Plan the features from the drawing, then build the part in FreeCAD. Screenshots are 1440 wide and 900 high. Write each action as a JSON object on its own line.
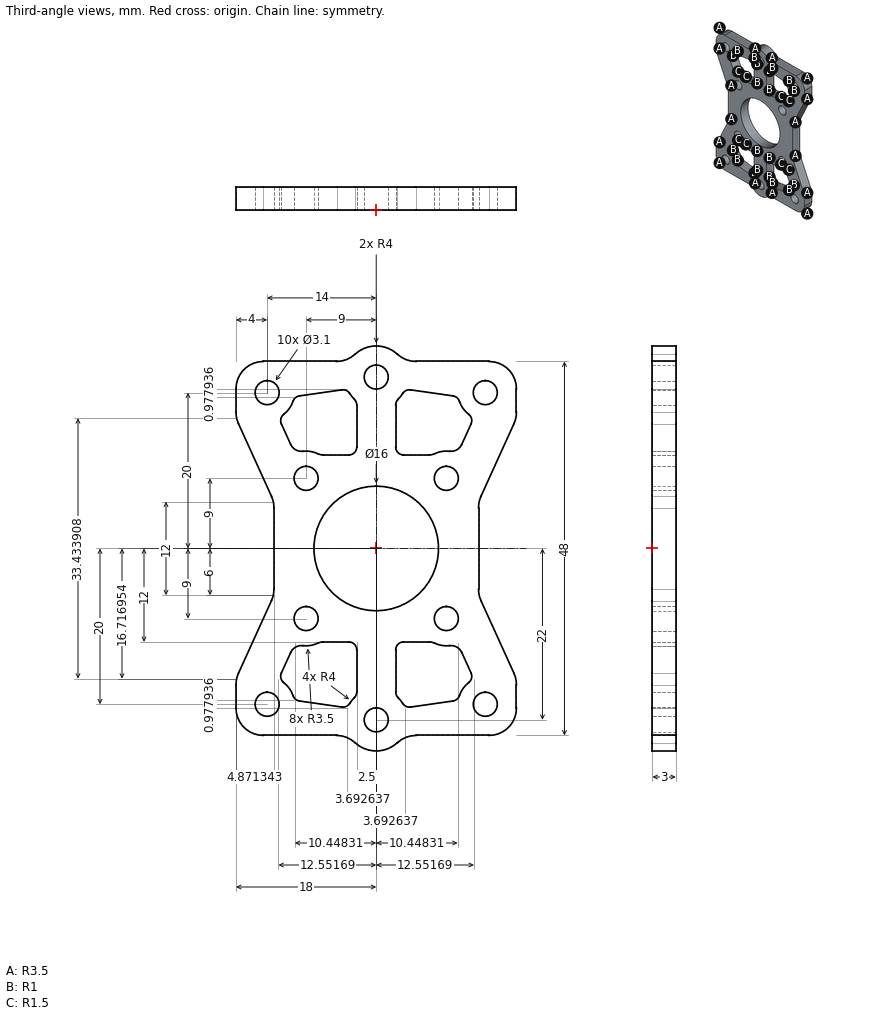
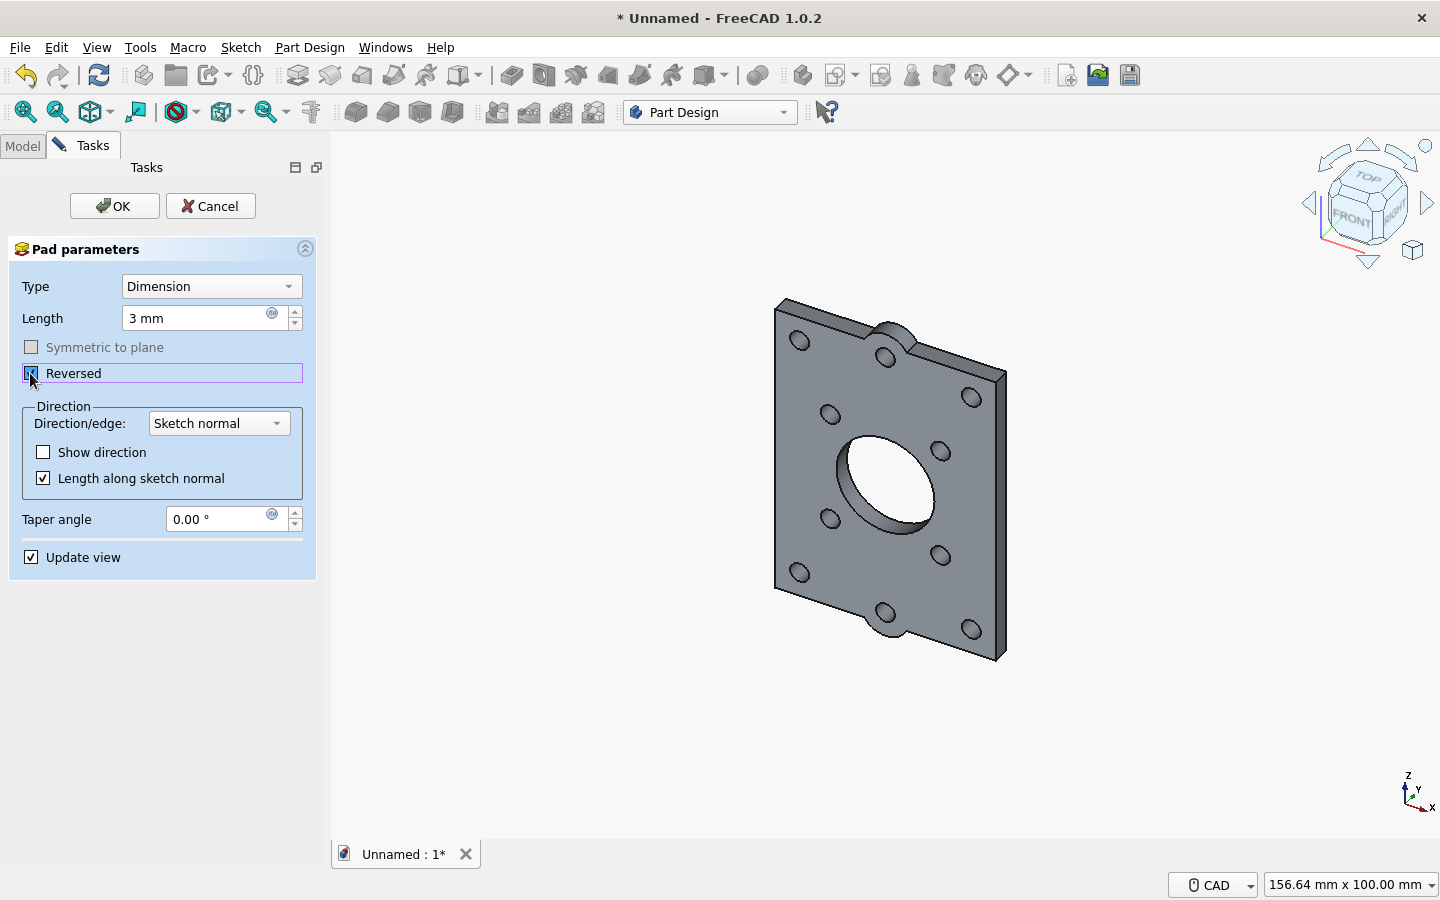
{"action": "left_click", "coordinate": [115, 206]}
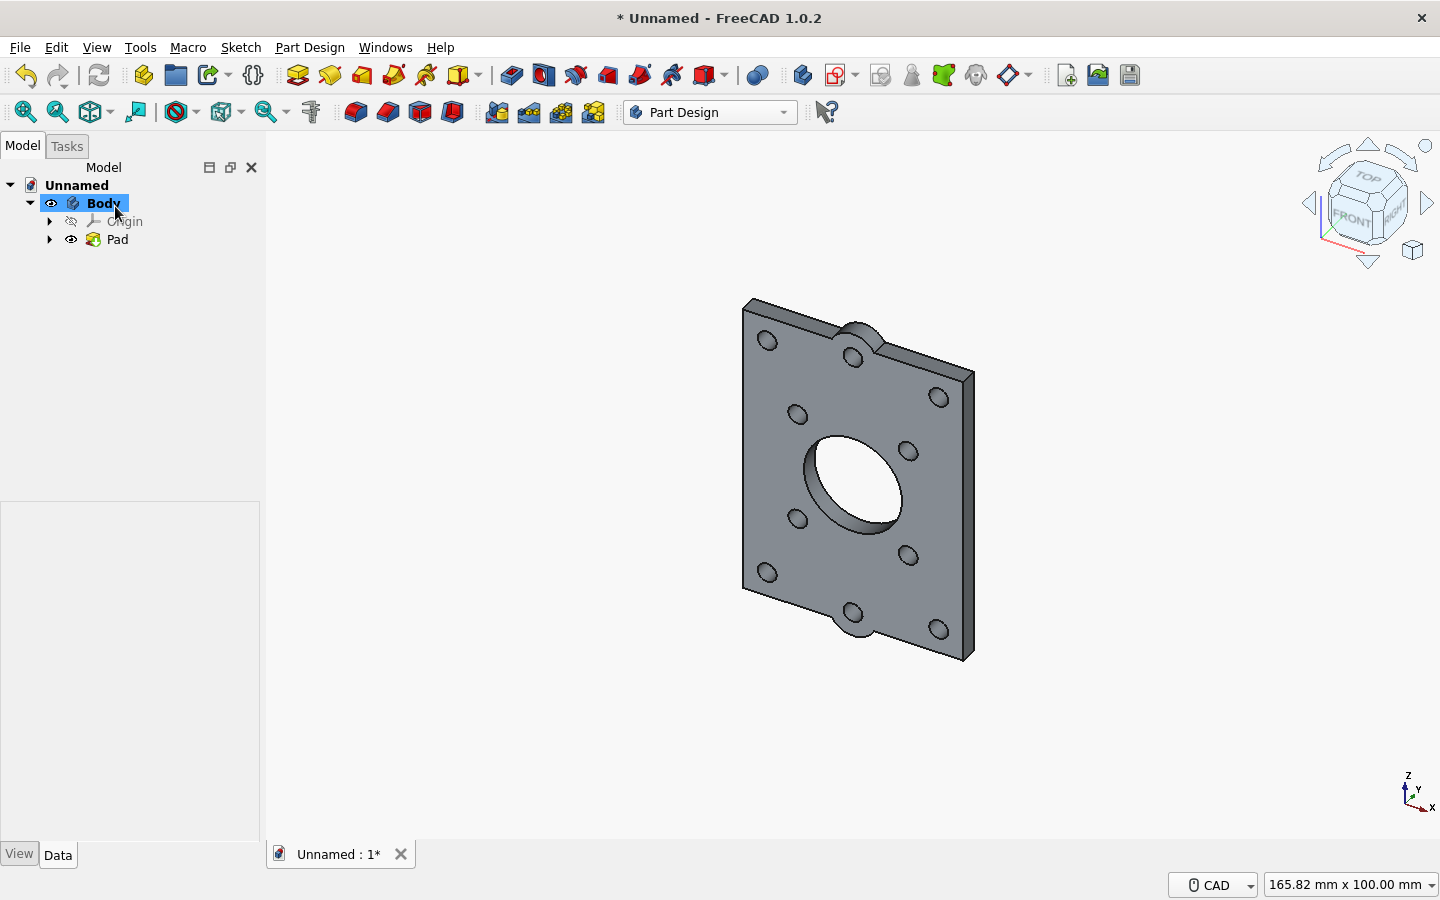
{"action": "key", "text": "4"}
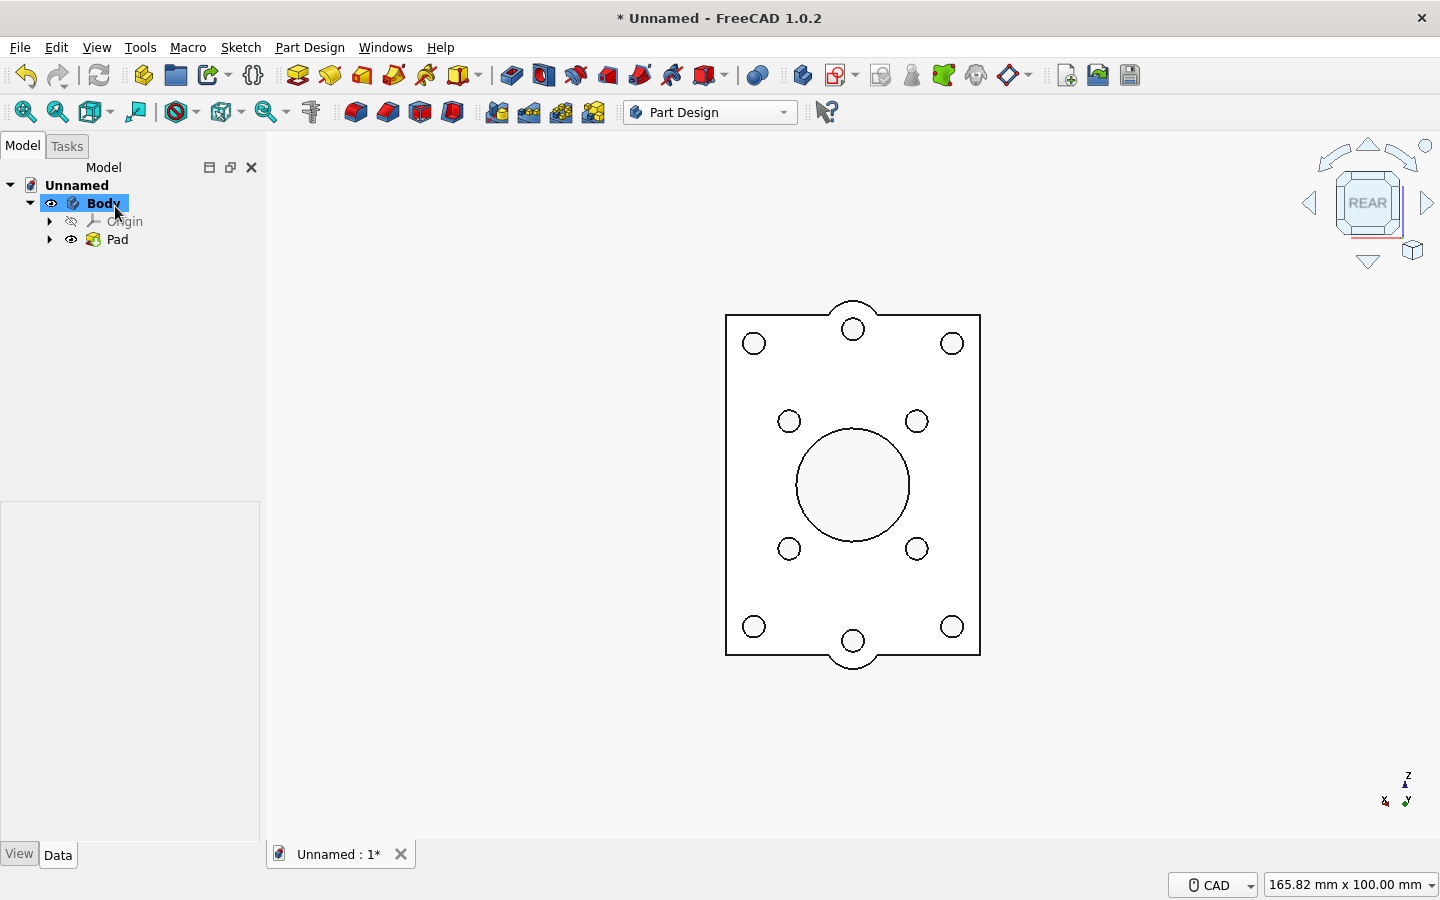
{"action": "left_click", "coordinate": [853, 379]}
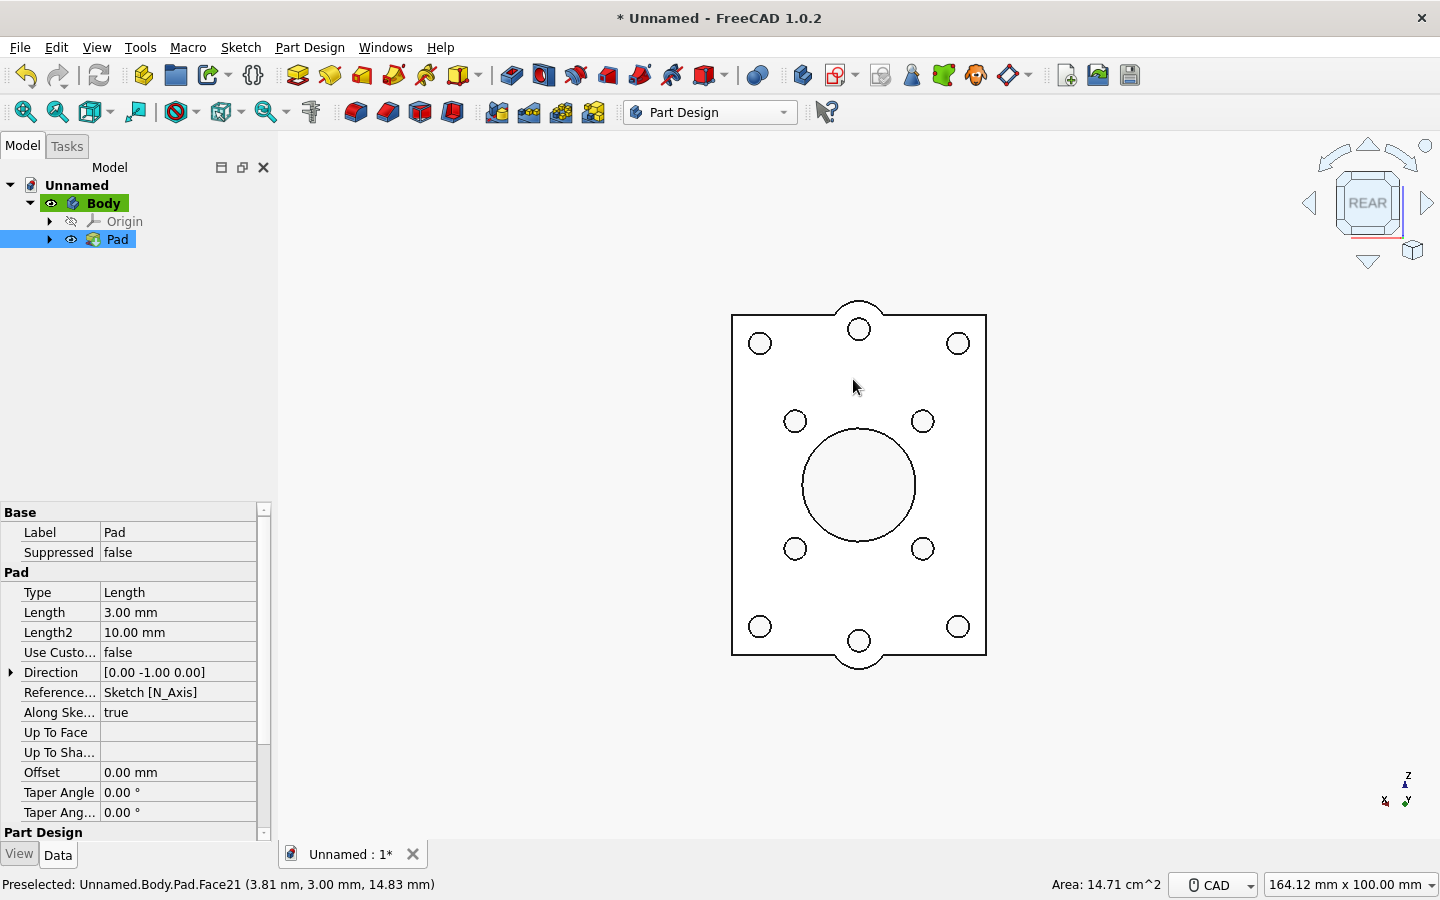
{"action": "left_click", "coordinate": [836, 76]}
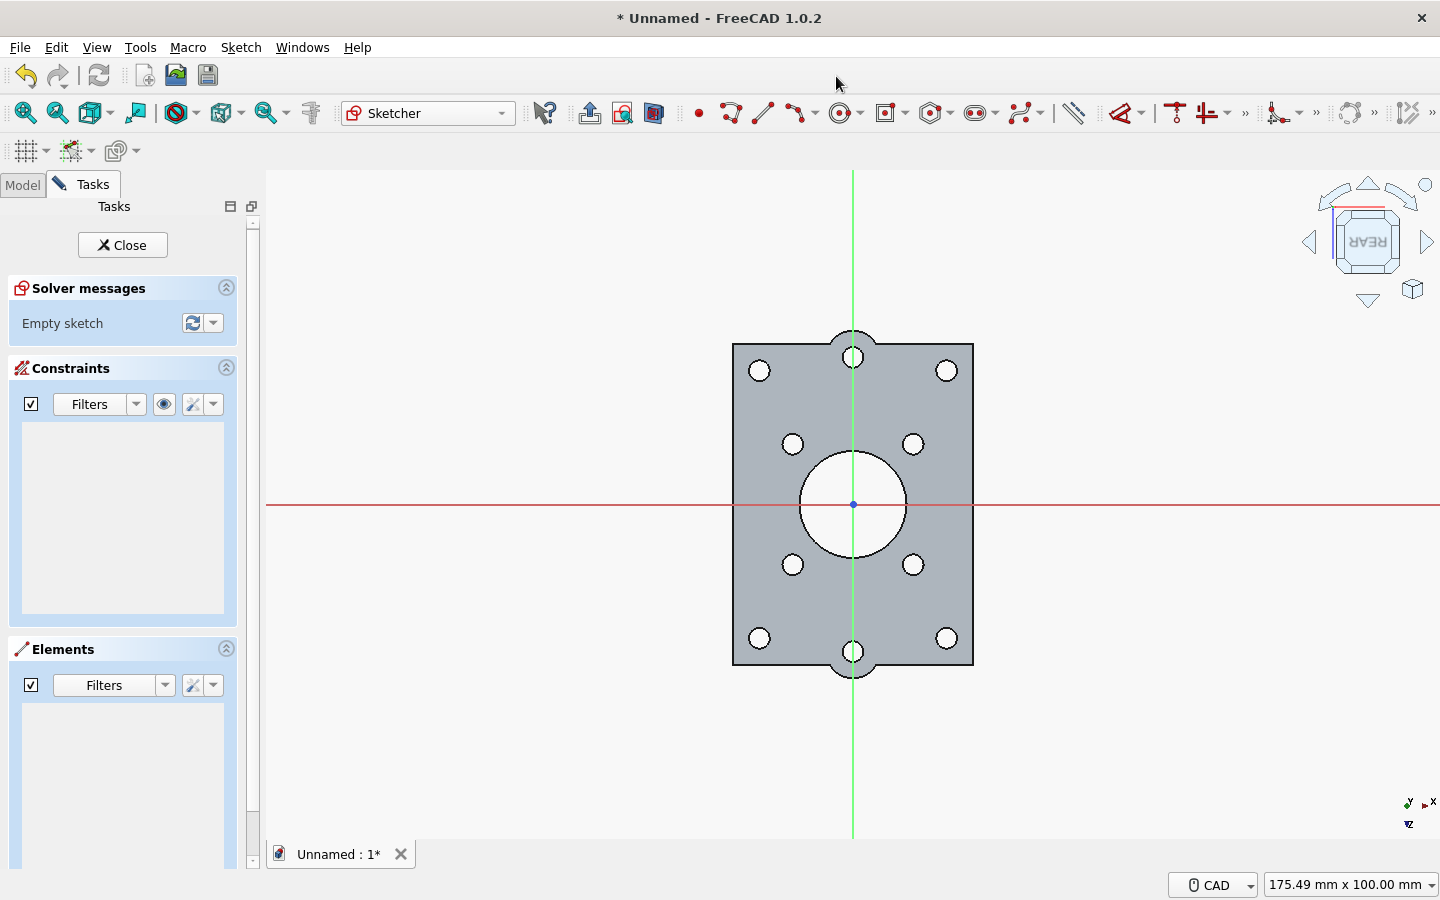
{"action": "scroll", "coordinate": [992, 505], "scroll_direction": "up", "scroll_amount": 2}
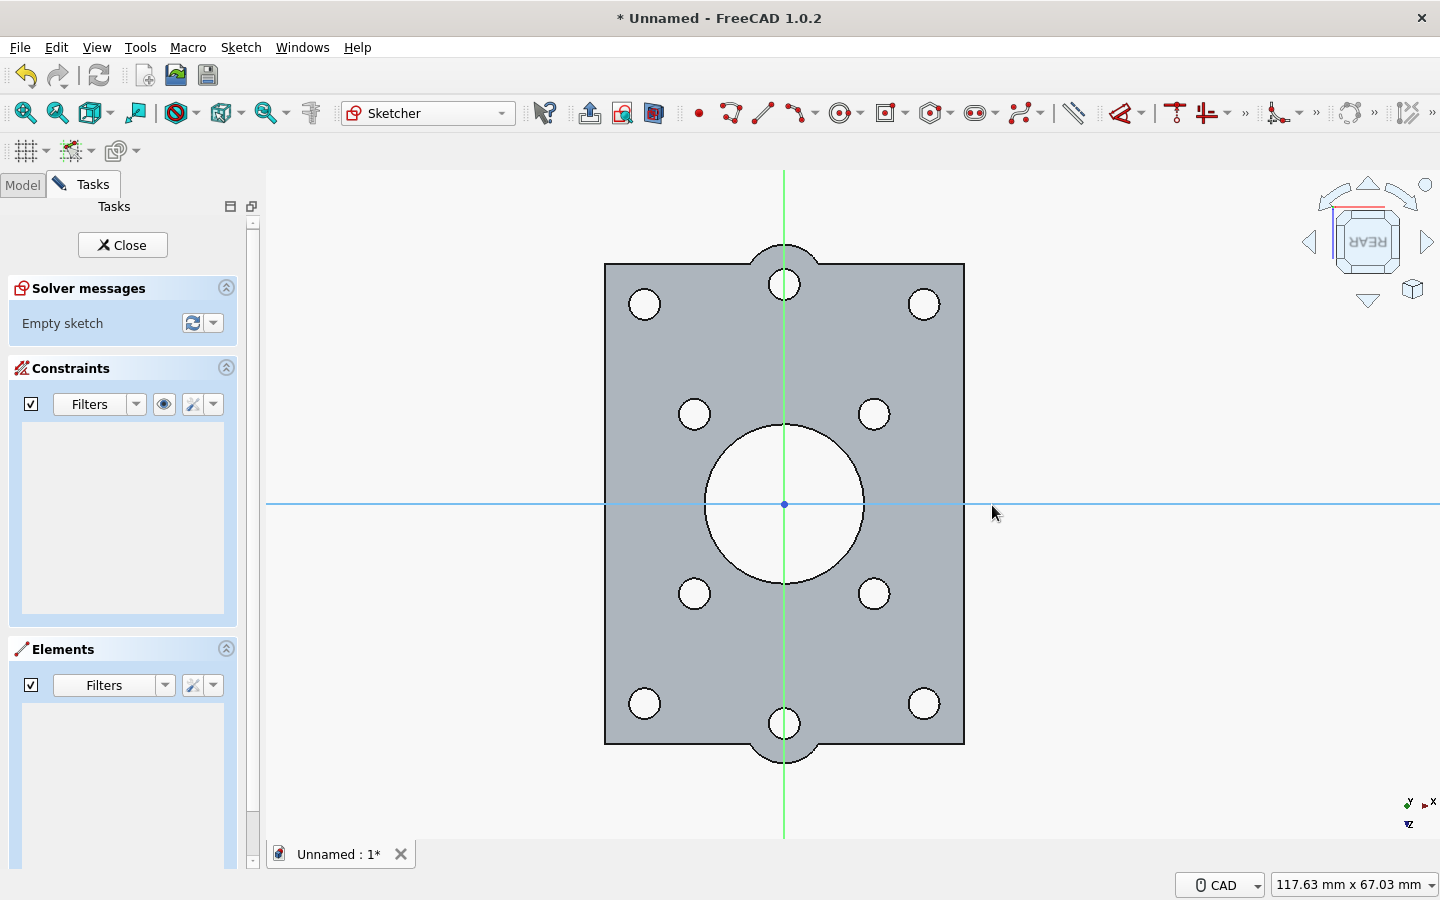
{"action": "key", "text": "g l"}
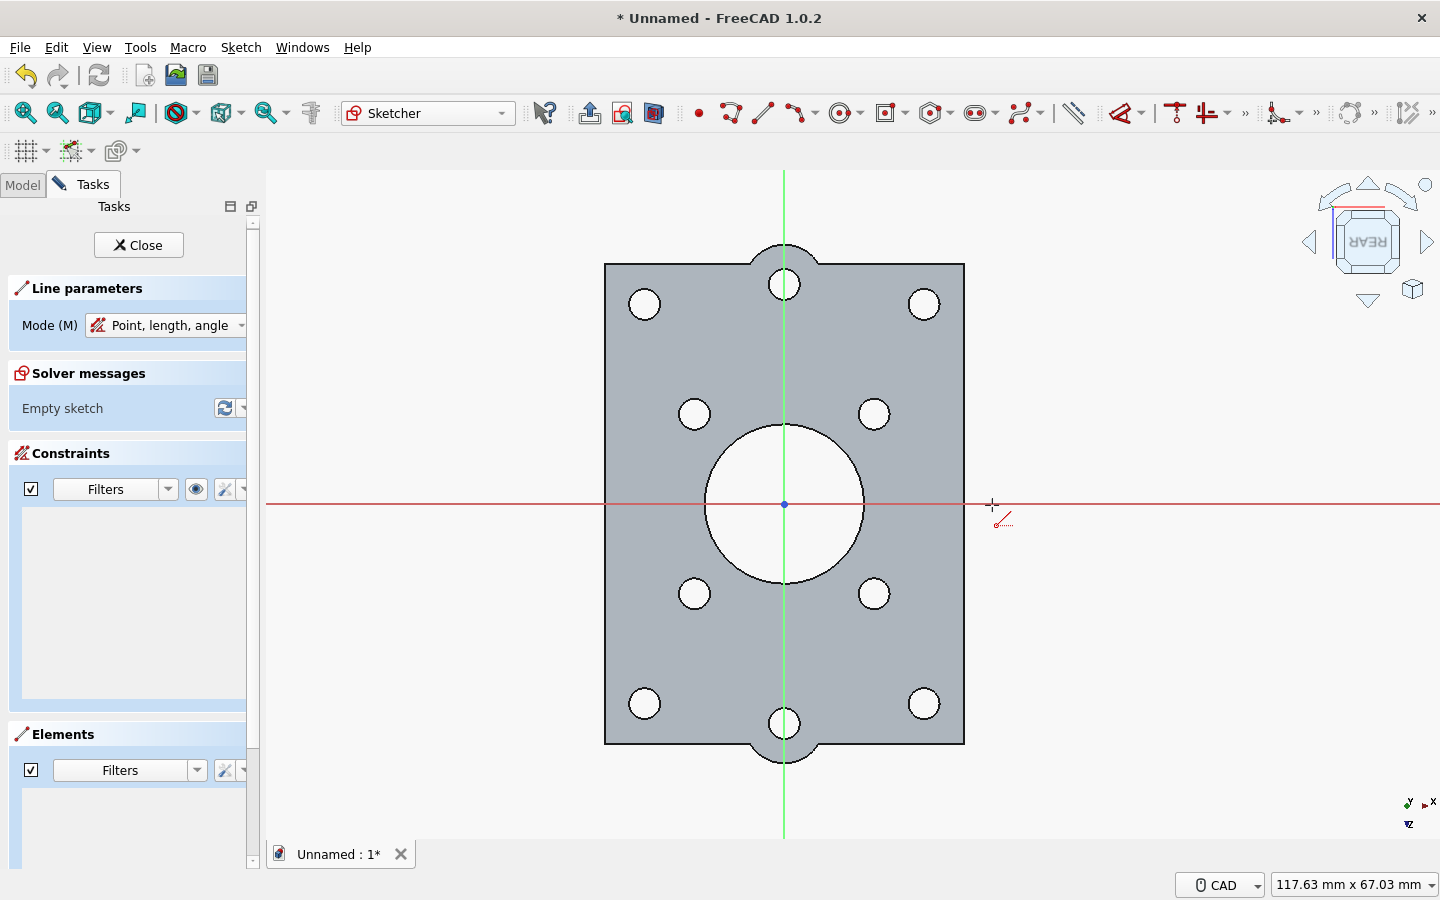
{"action": "left_click", "coordinate": [659, 336]}
{"action": "left_click", "coordinate": [680, 382]}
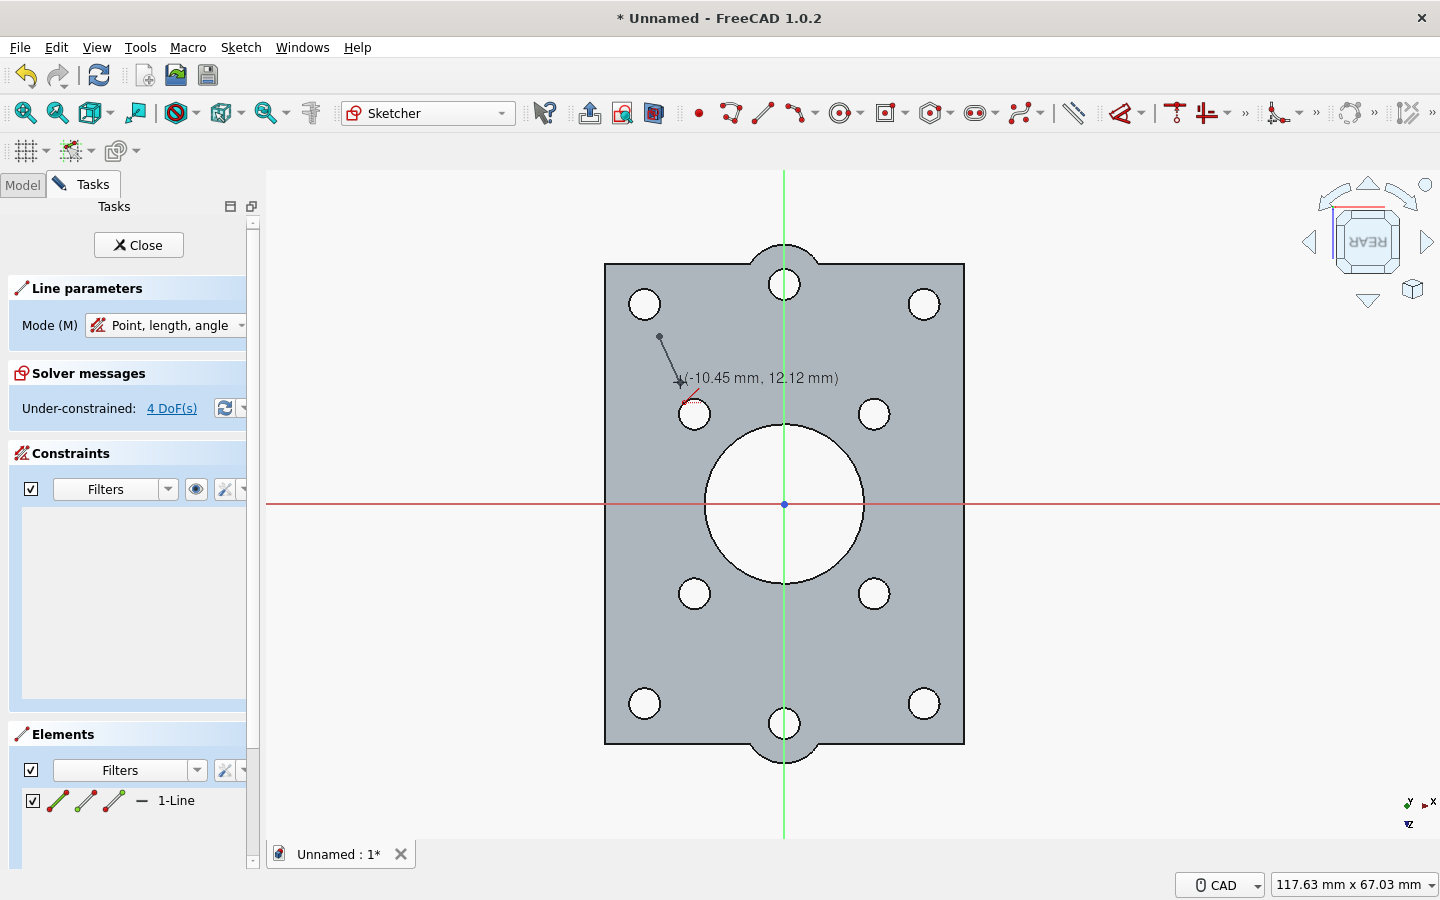
{"action": "left_click", "coordinate": [732, 114]}